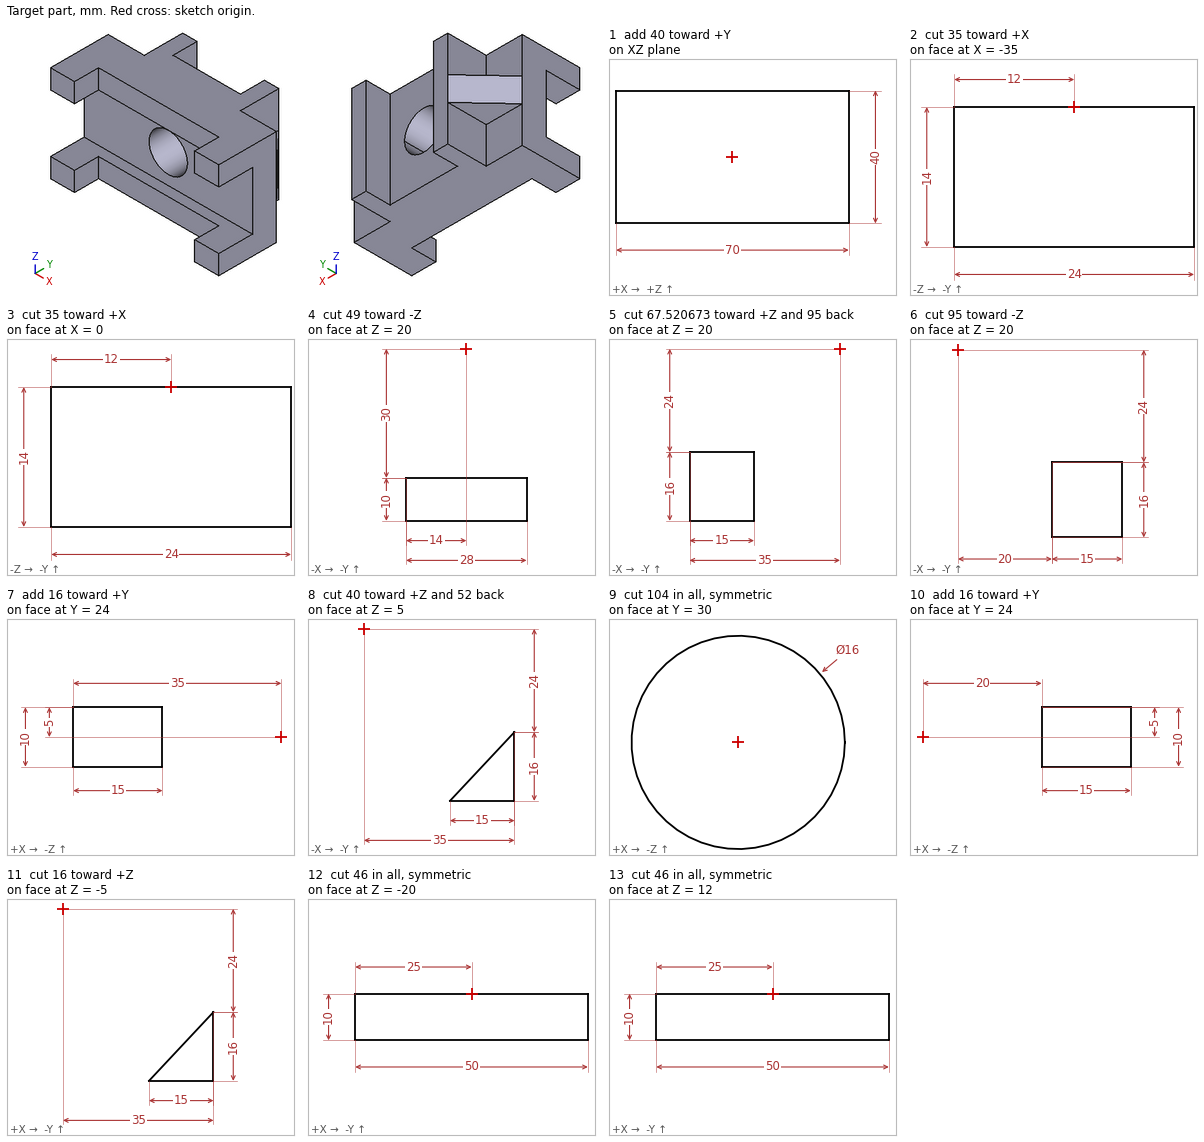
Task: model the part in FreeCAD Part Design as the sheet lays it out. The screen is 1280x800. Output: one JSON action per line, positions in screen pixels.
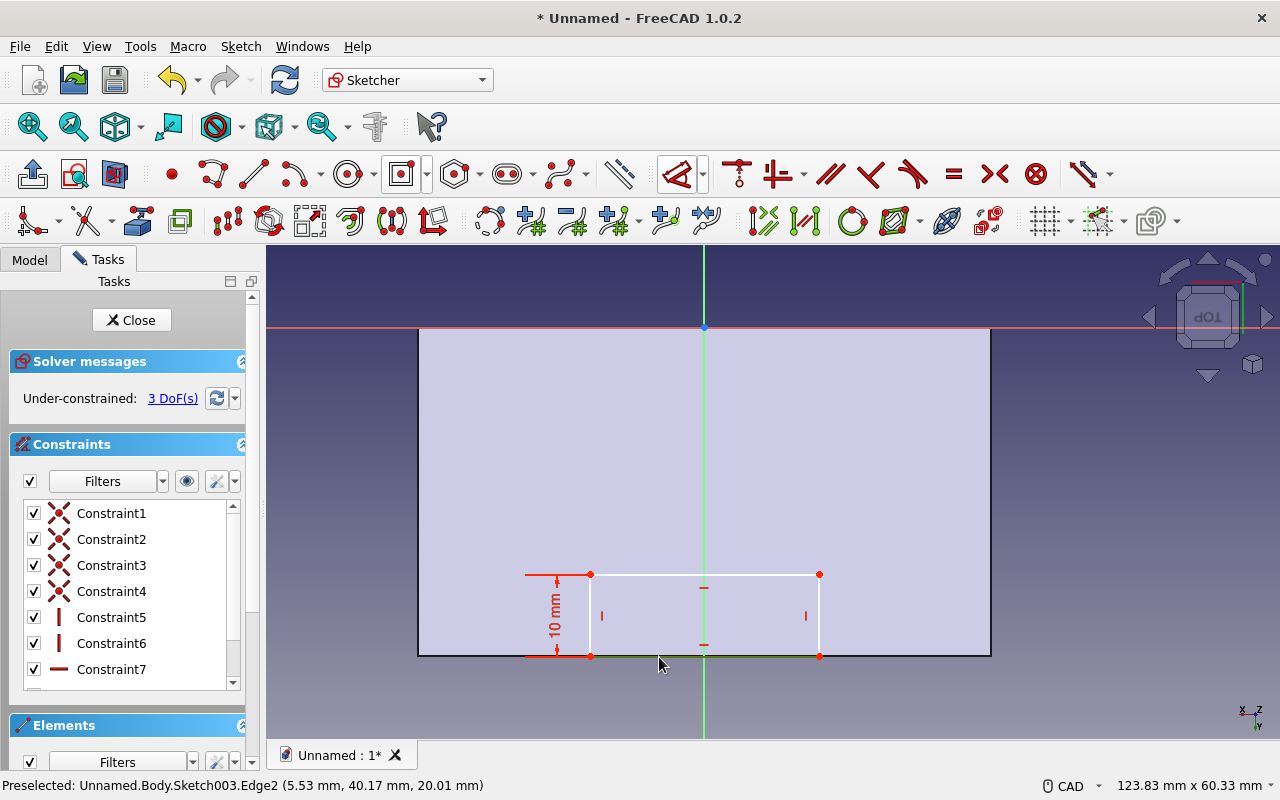
{"action": "key", "text": "l"}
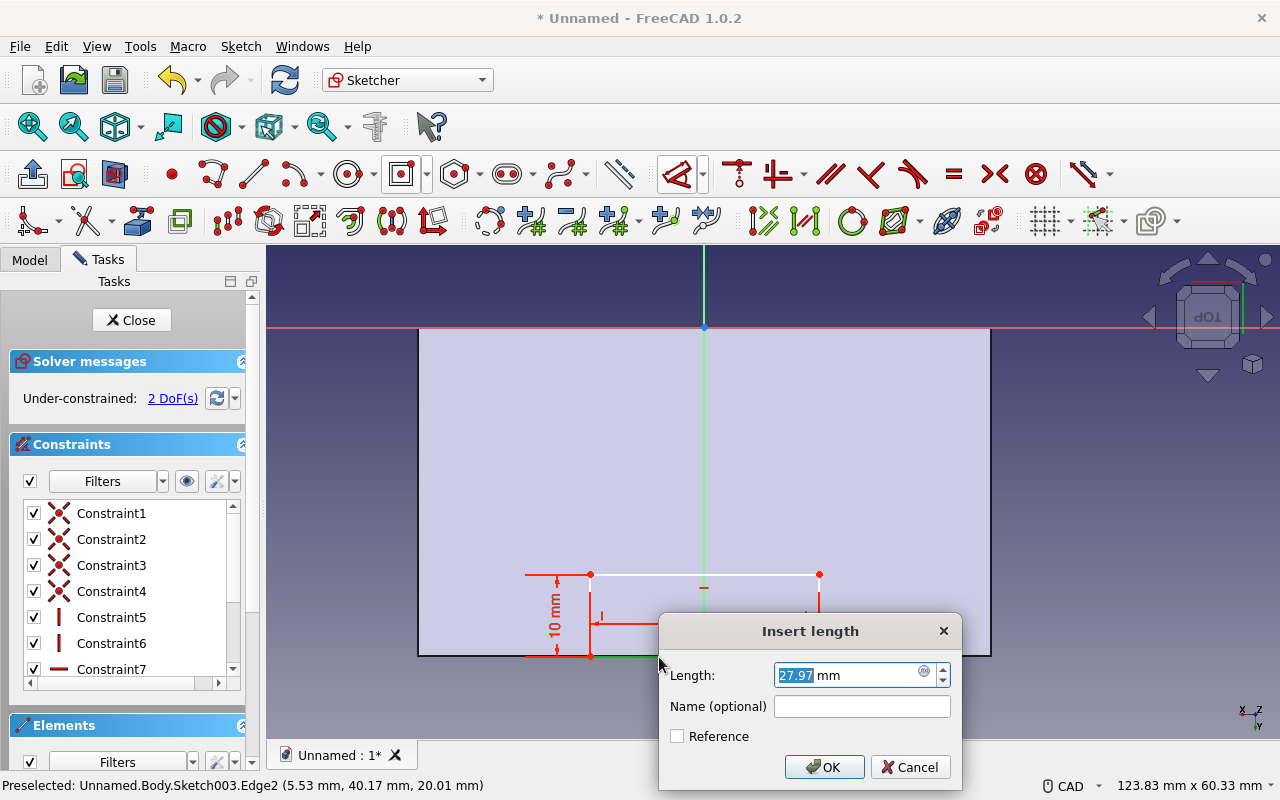
{"action": "type", "text": "28"}
{"action": "key", "text": "Return"}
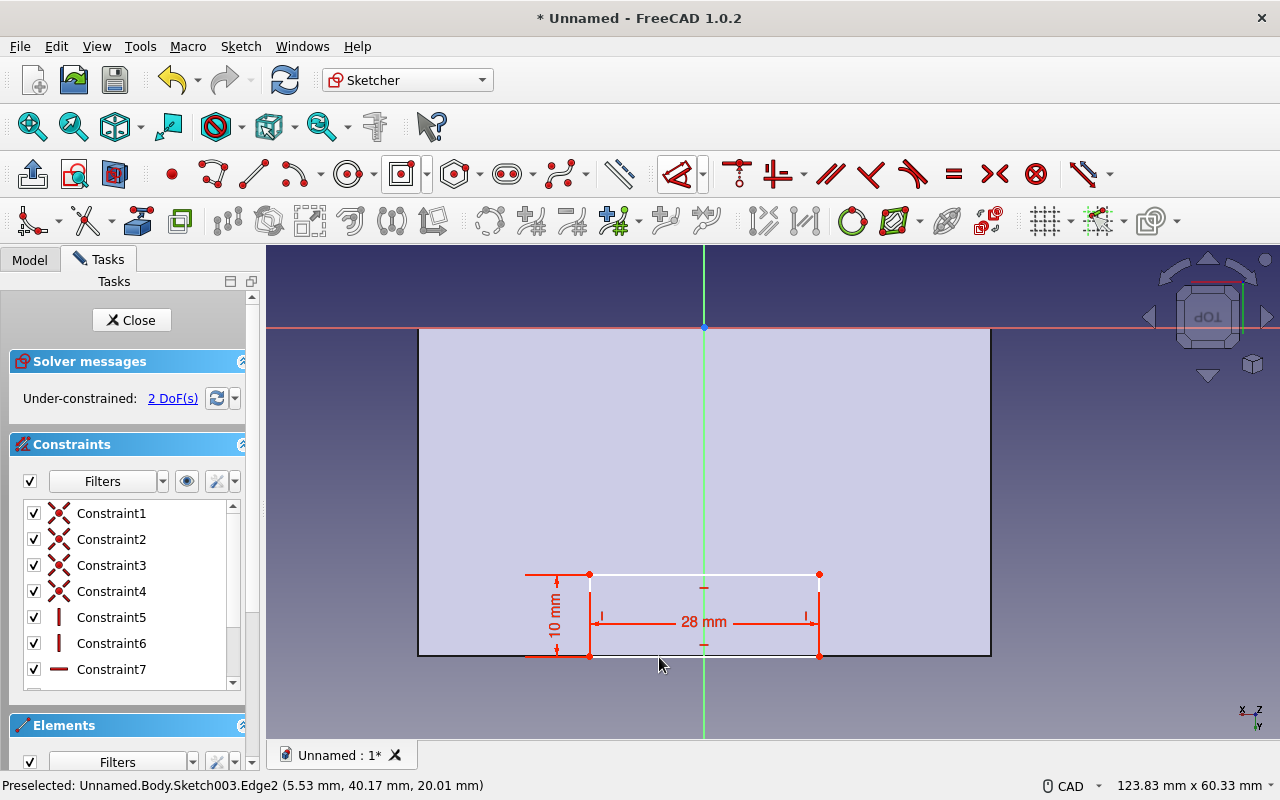
{"action": "left_click", "coordinate": [590, 575]}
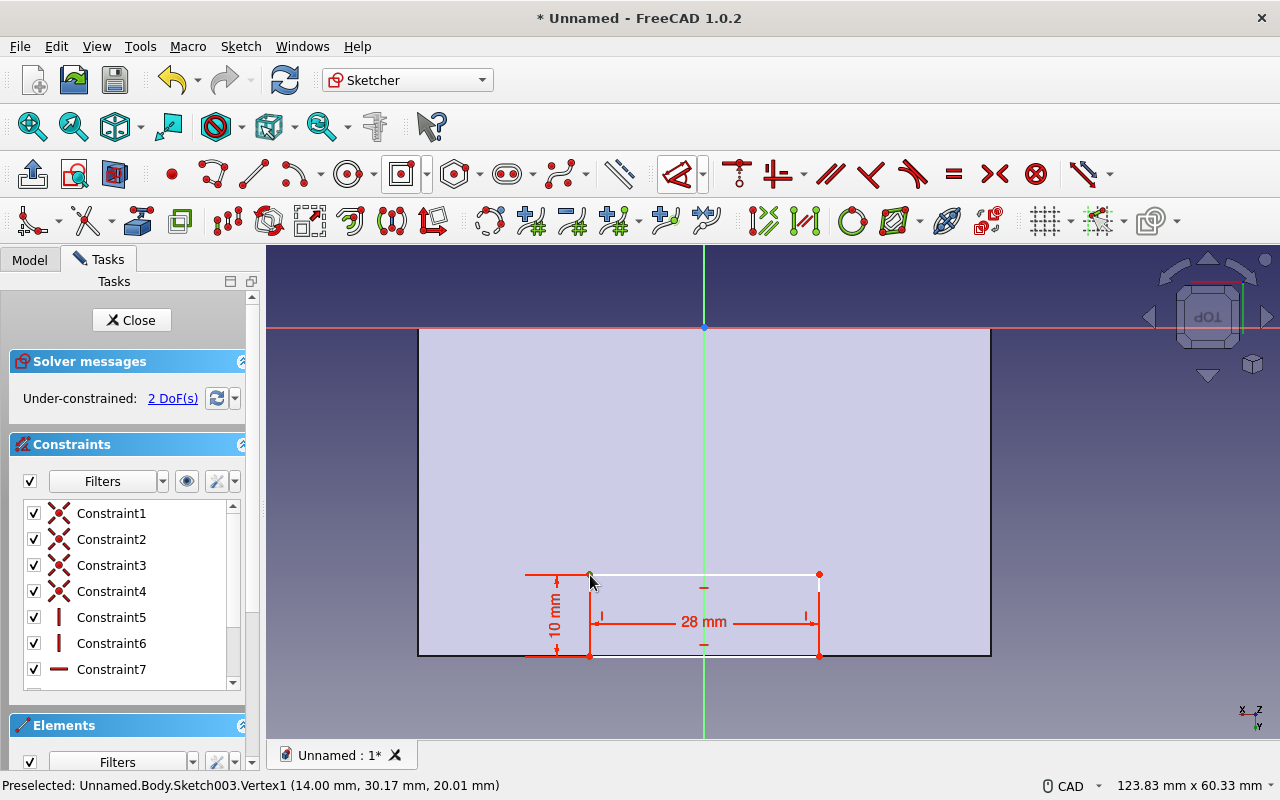
{"action": "key", "text": "l"}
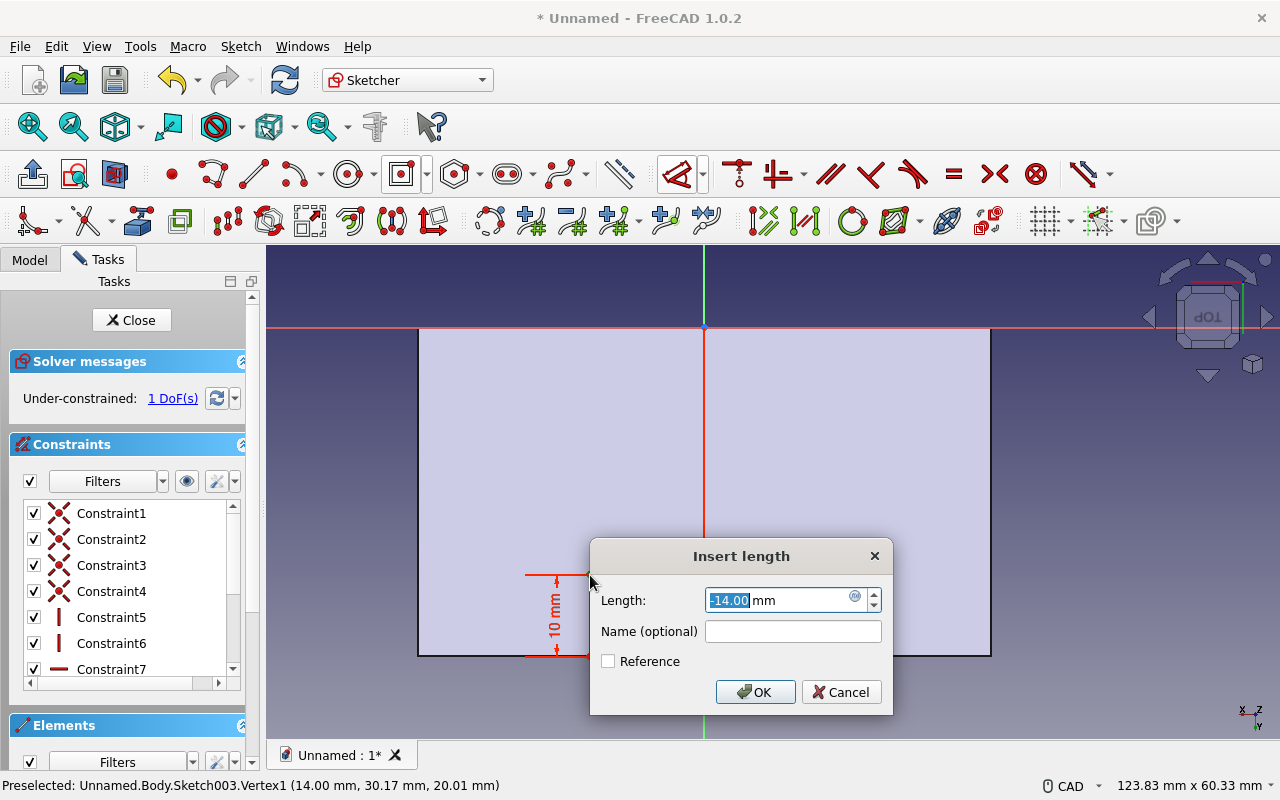
{"action": "type", "text": "-14"}
{"action": "key", "text": "Return"}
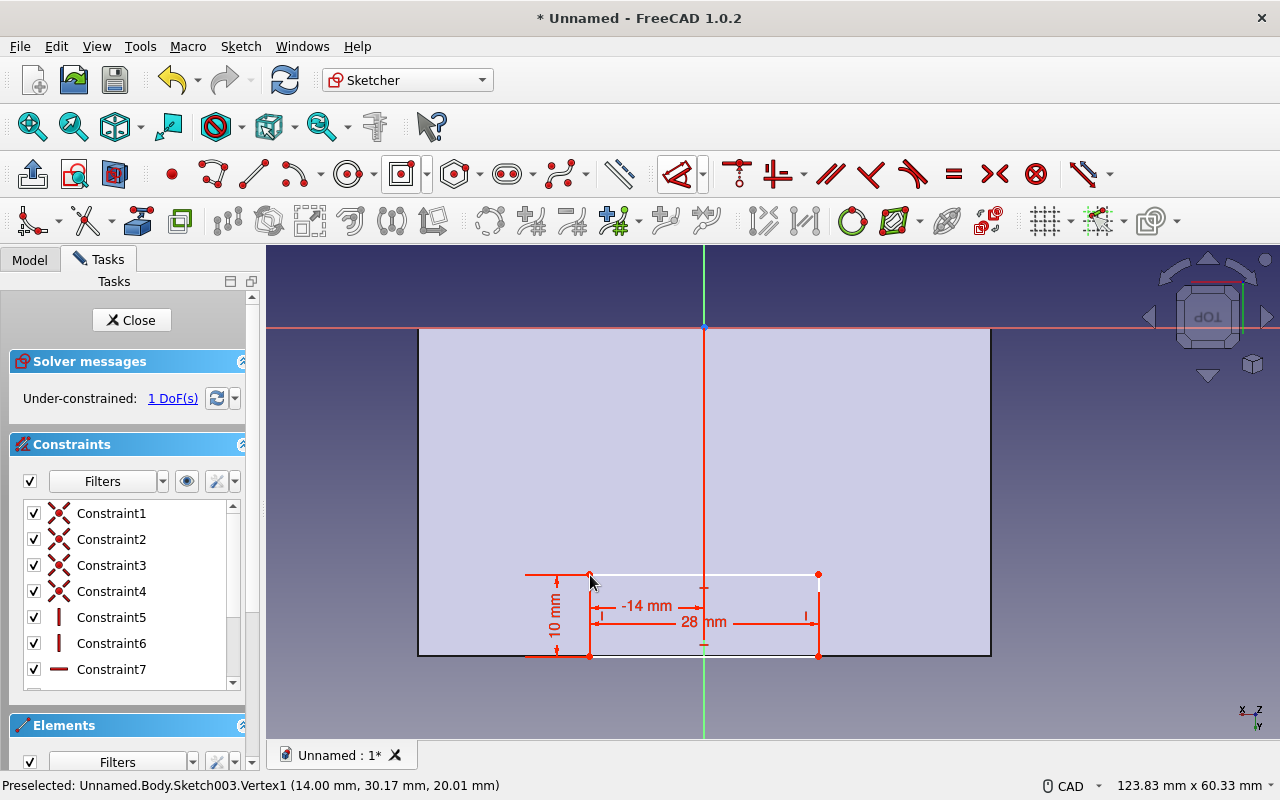
{"action": "left_click", "coordinate": [590, 575]}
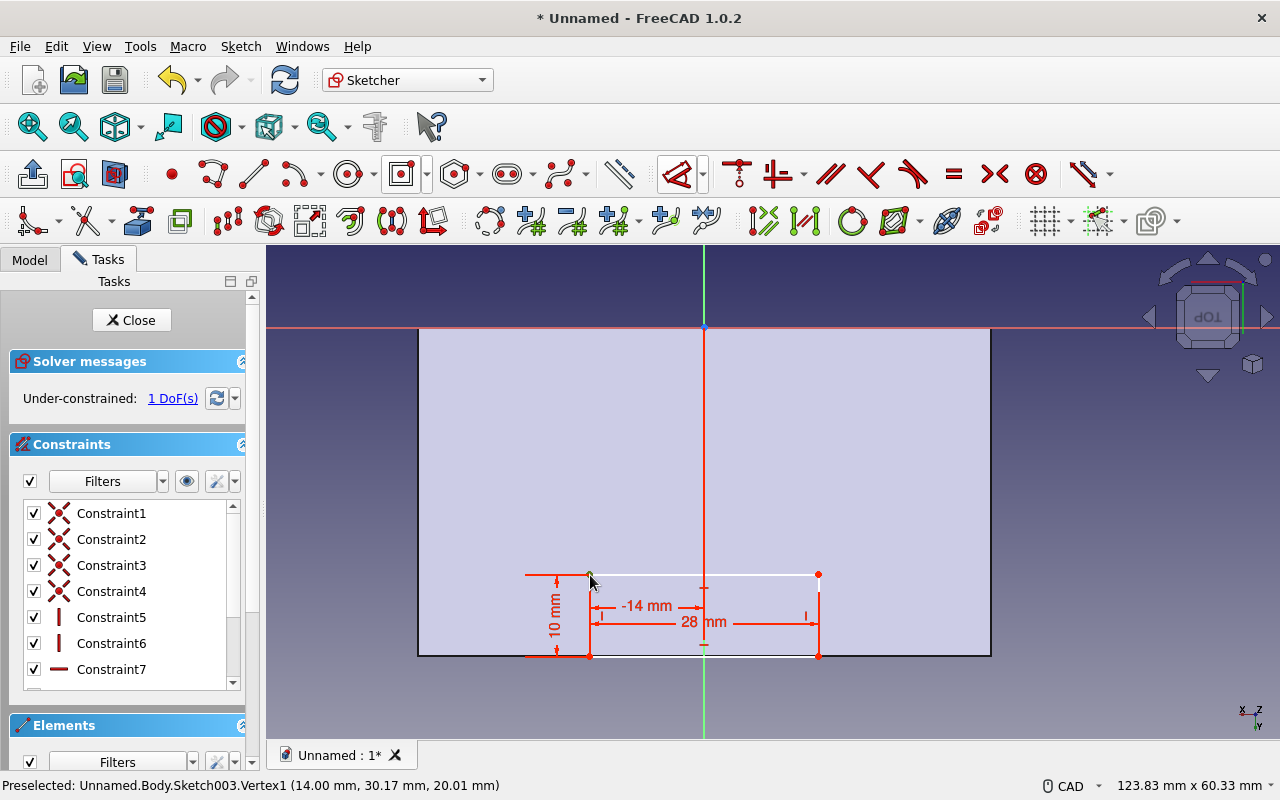
{"action": "key", "text": "i"}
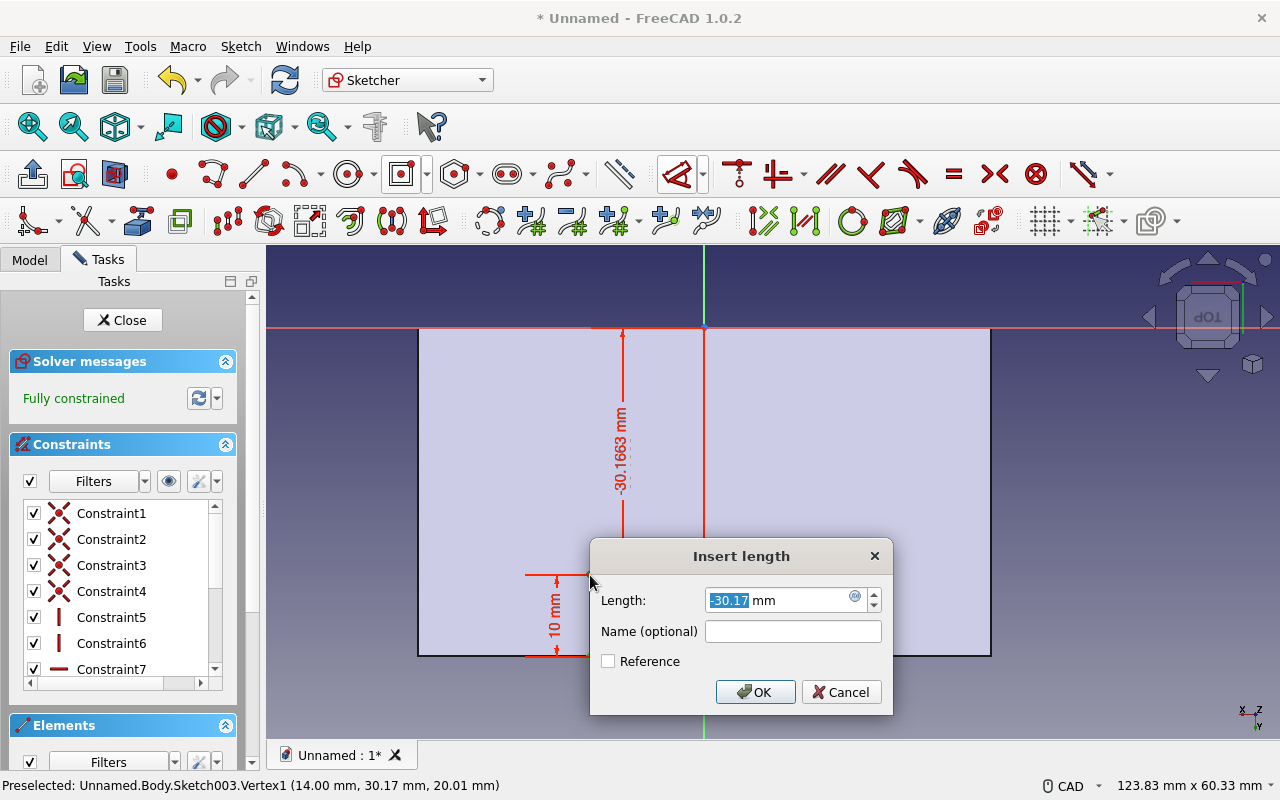
{"action": "type", "text": "-30"}
{"action": "key", "text": "Return"}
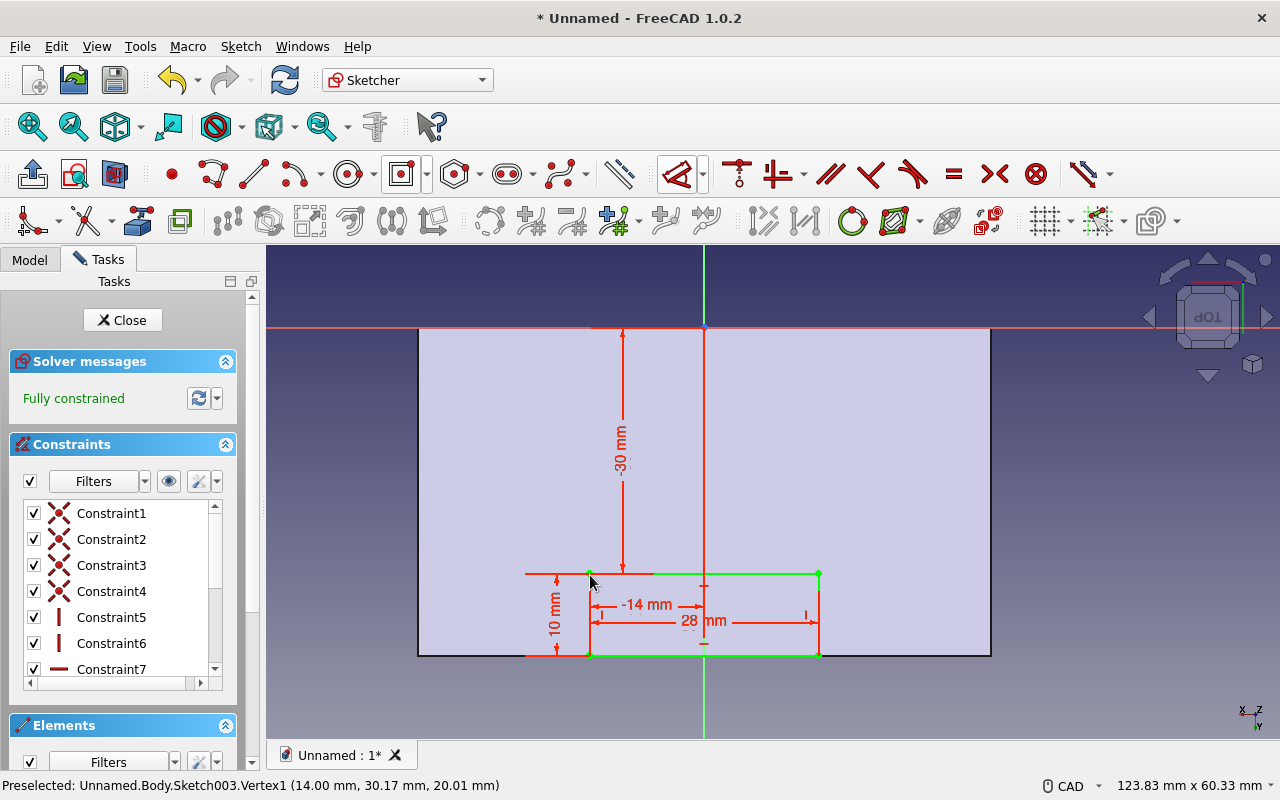
{"action": "left_click", "coordinate": [123, 320]}